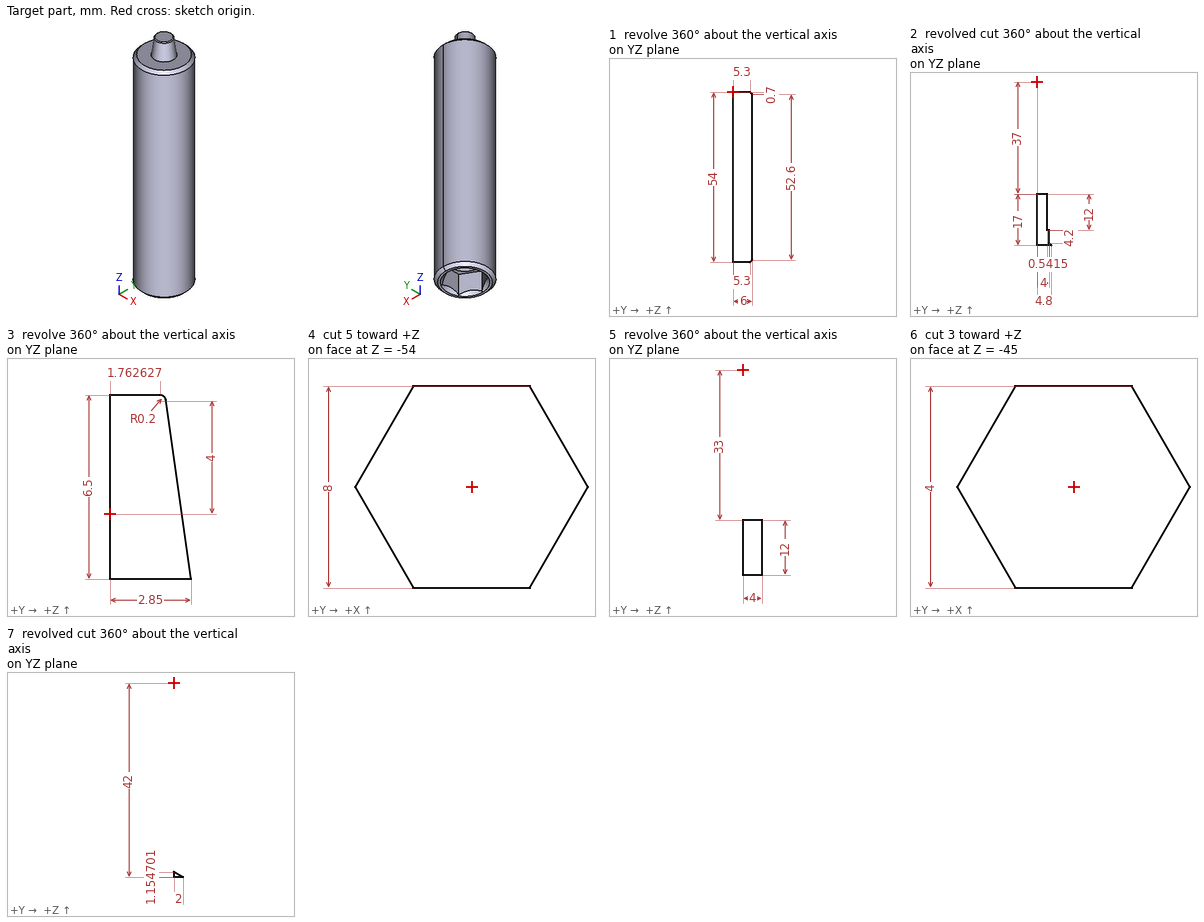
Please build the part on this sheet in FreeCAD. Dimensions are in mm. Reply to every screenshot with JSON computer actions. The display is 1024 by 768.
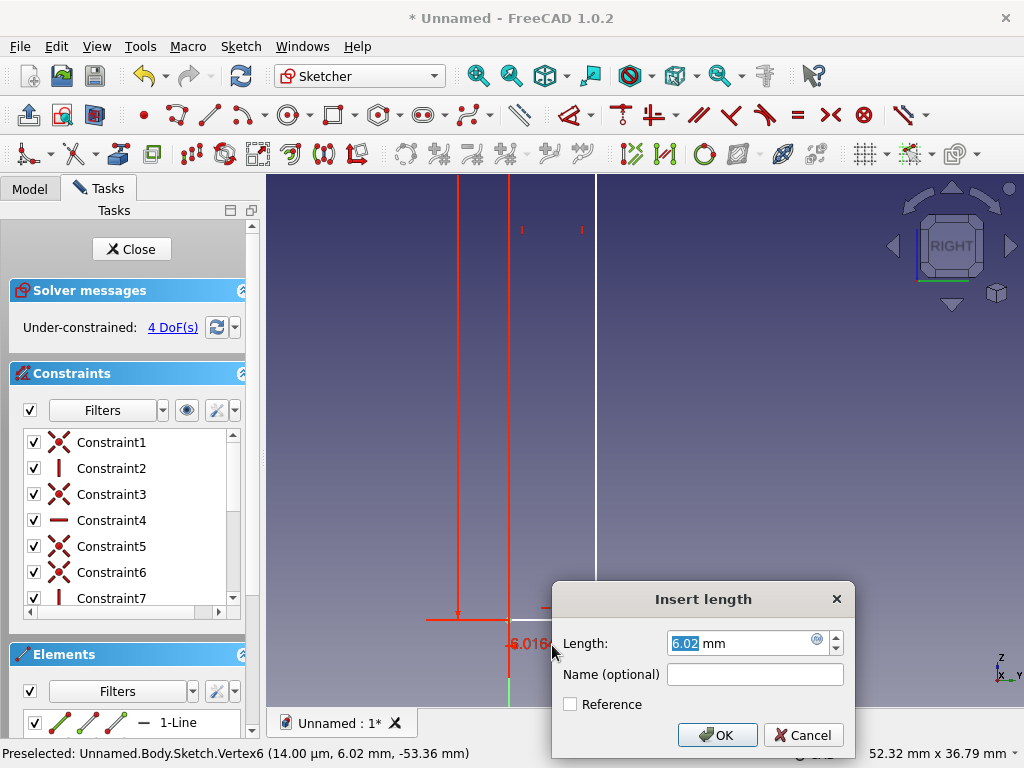
{"action": "type", "text": "6"}
{"action": "key", "text": "Return"}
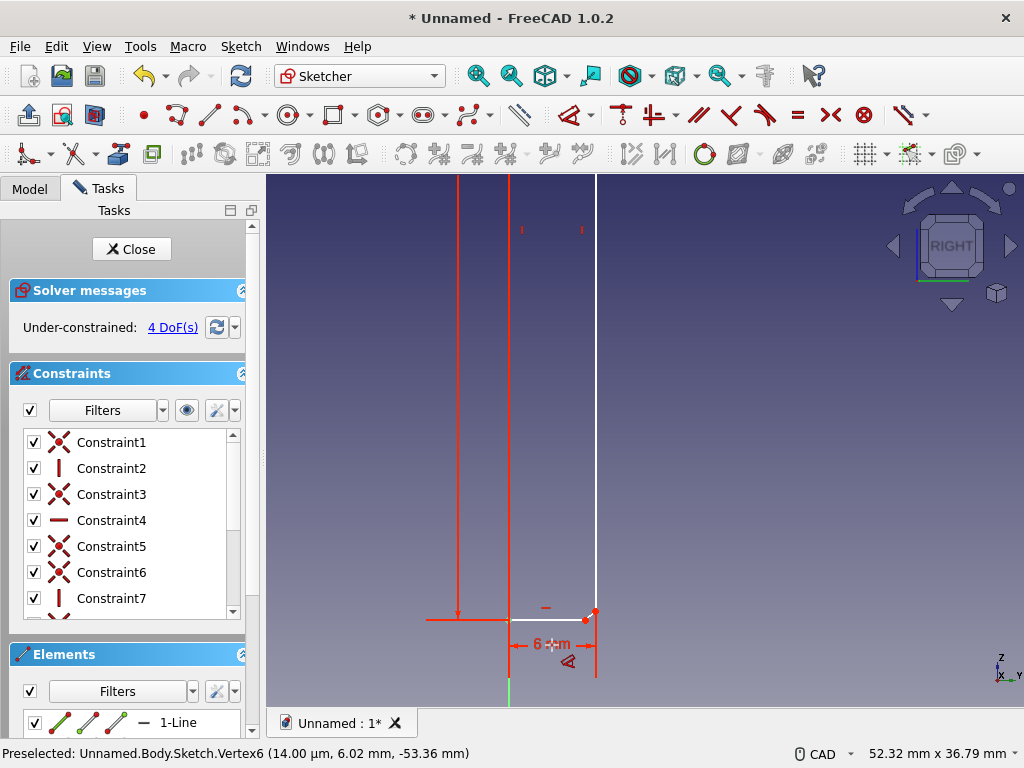
{"action": "left_click", "coordinate": [532, 620]}
{"action": "left_click", "coordinate": [547, 586]}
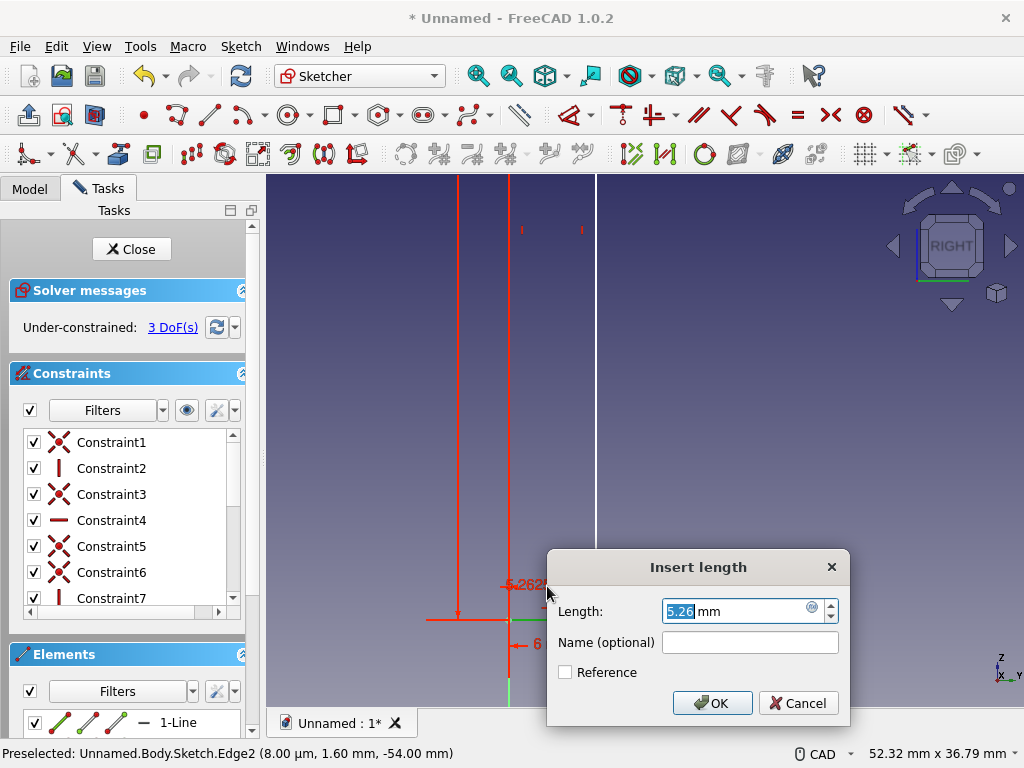
{"action": "type", "text": "5.3"}
{"action": "key", "text": "Return"}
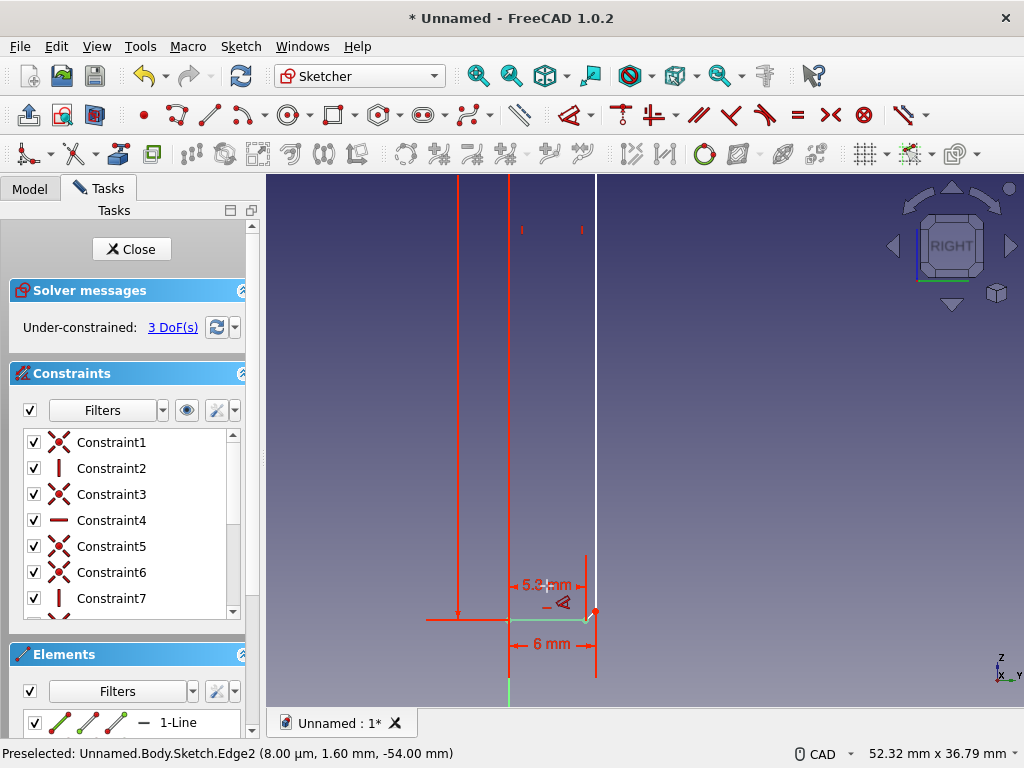
{"action": "scroll", "coordinate": [596, 613], "scroll_direction": "down", "scroll_amount": 4}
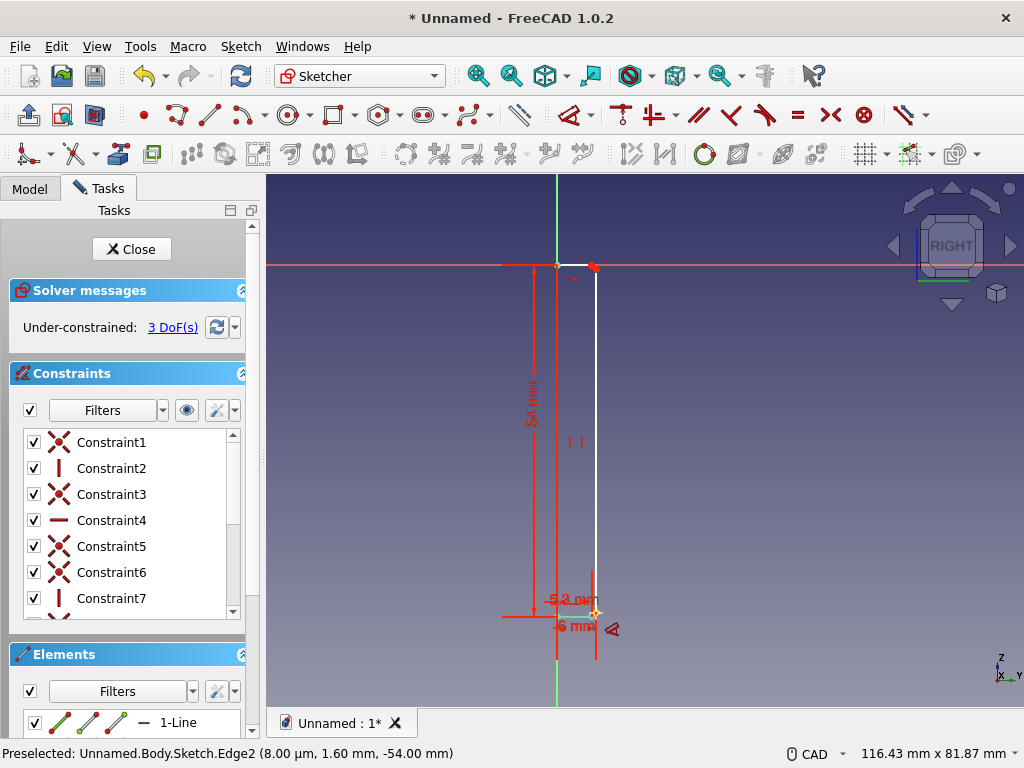
{"action": "scroll", "coordinate": [581, 265], "scroll_direction": "up", "scroll_amount": 2}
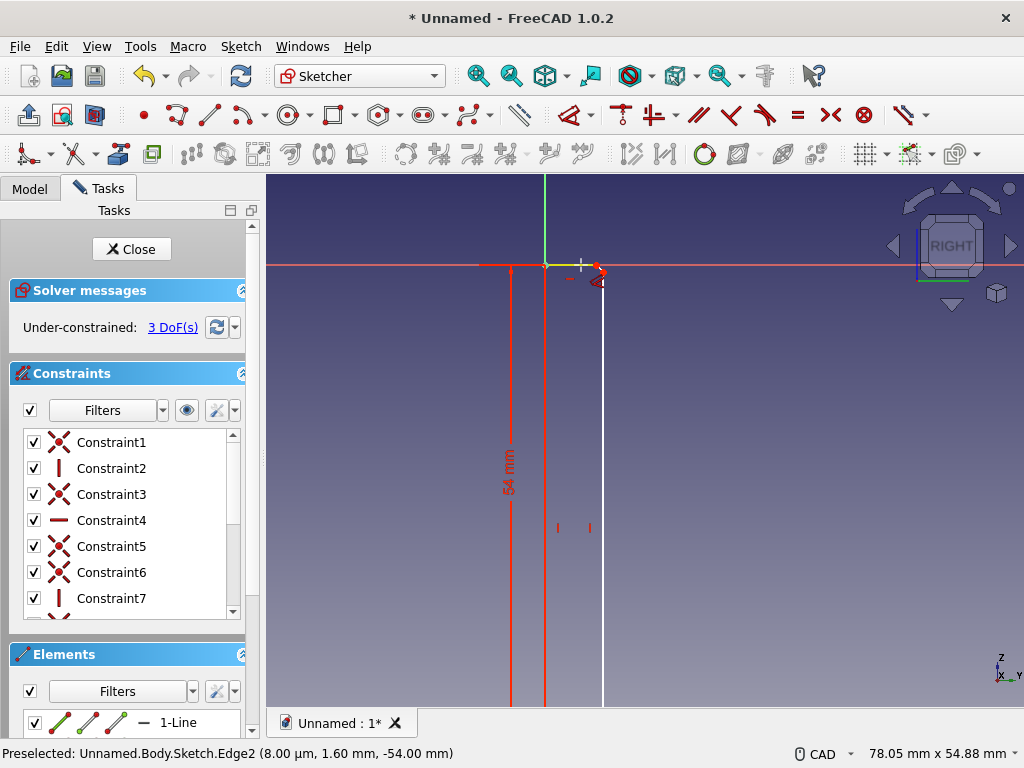
{"action": "left_click", "coordinate": [581, 265]}
{"action": "left_click", "coordinate": [571, 231]}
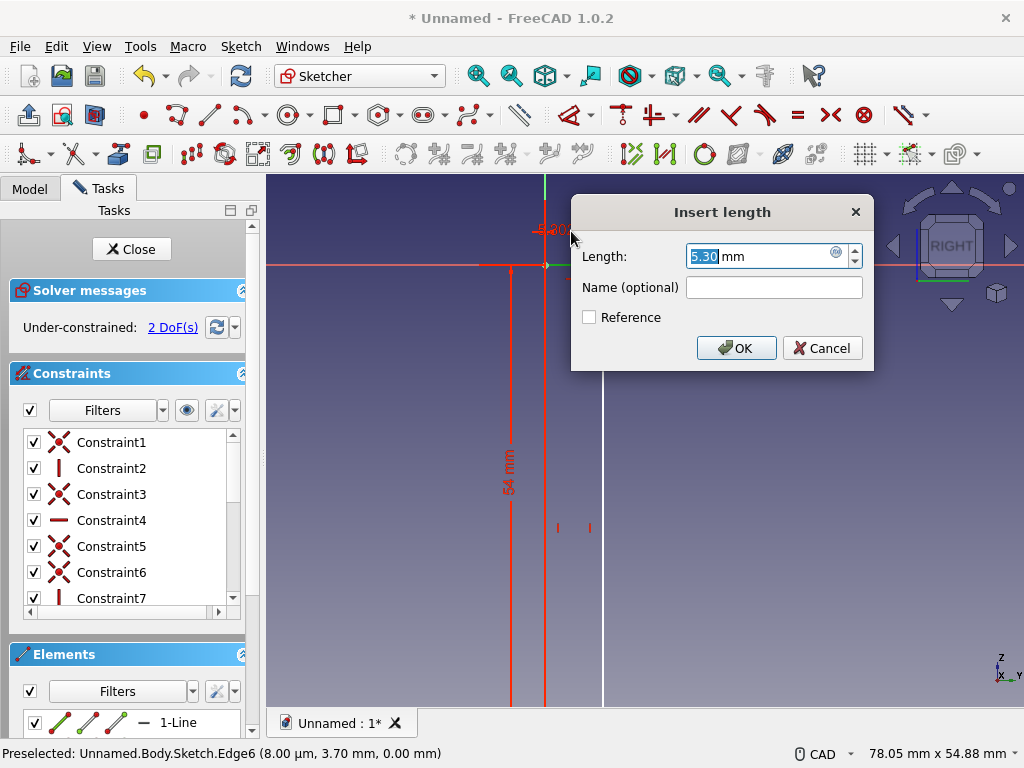
{"action": "type", "text": "5.3"}
{"action": "key", "text": "Return"}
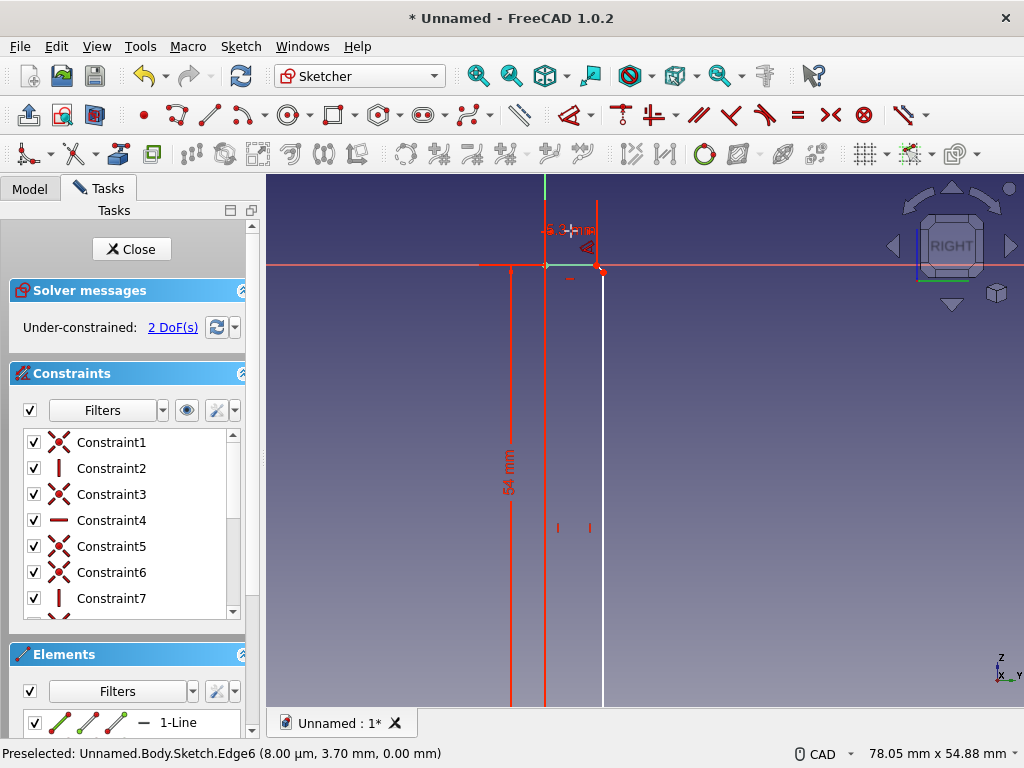
{"action": "left_click", "coordinate": [603, 630]}
{"action": "left_click", "coordinate": [637, 476]}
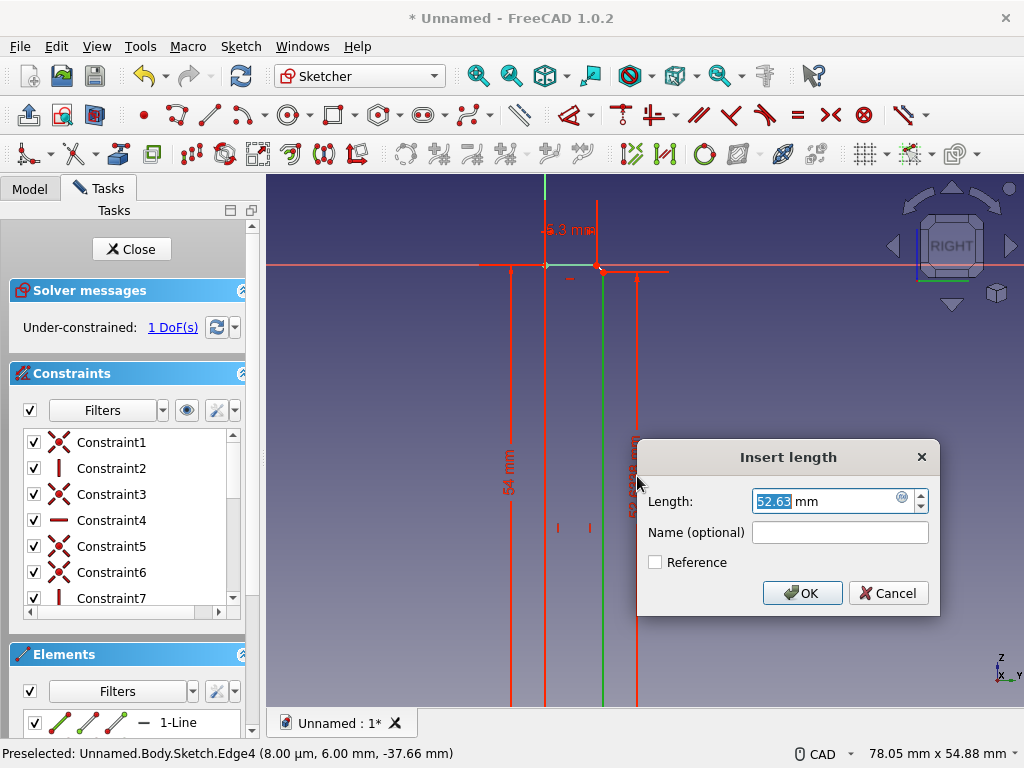
{"action": "type", "text": "52.6"}
{"action": "key", "text": "Return"}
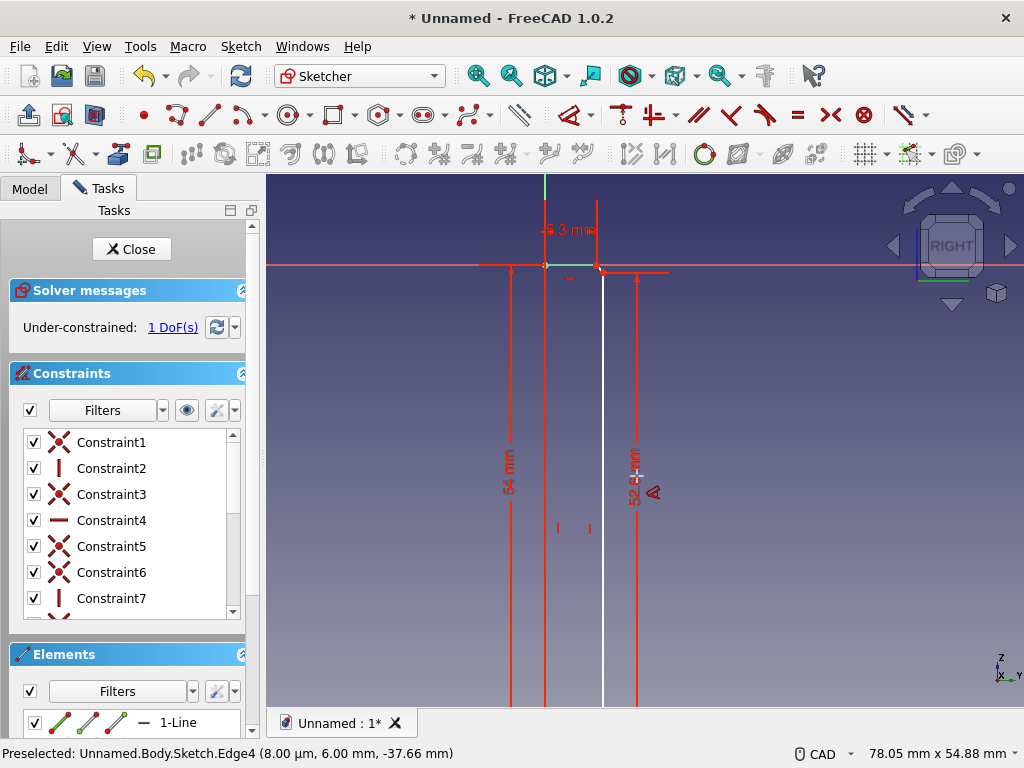
{"action": "scroll", "coordinate": [603, 273], "scroll_direction": "up", "scroll_amount": 9}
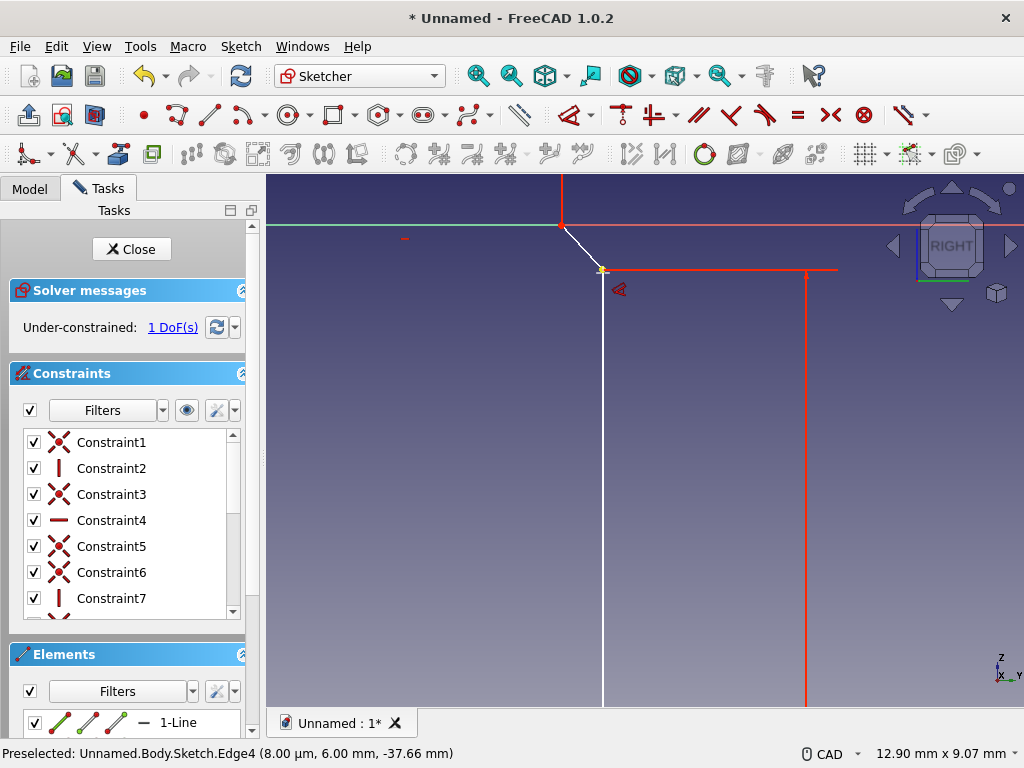
{"action": "left_click", "coordinate": [603, 270]}
{"action": "left_click", "coordinate": [637, 247]}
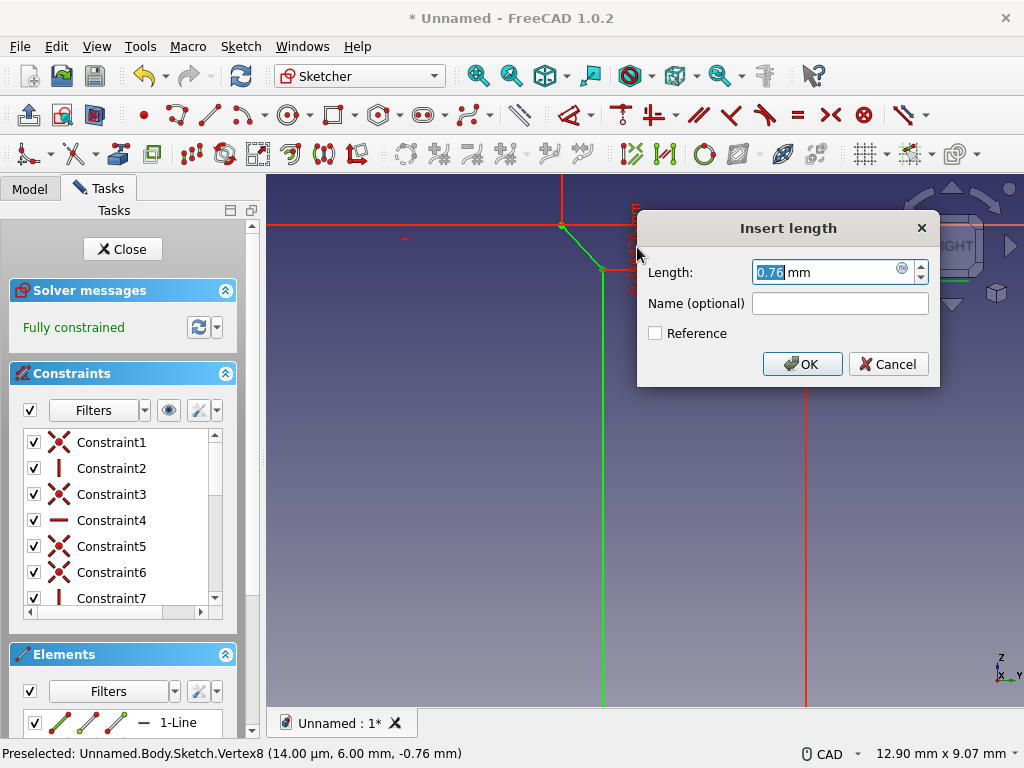
{"action": "type", "text": "0.7"}
{"action": "key", "text": "Return"}
{"action": "key", "text": "Escape"}